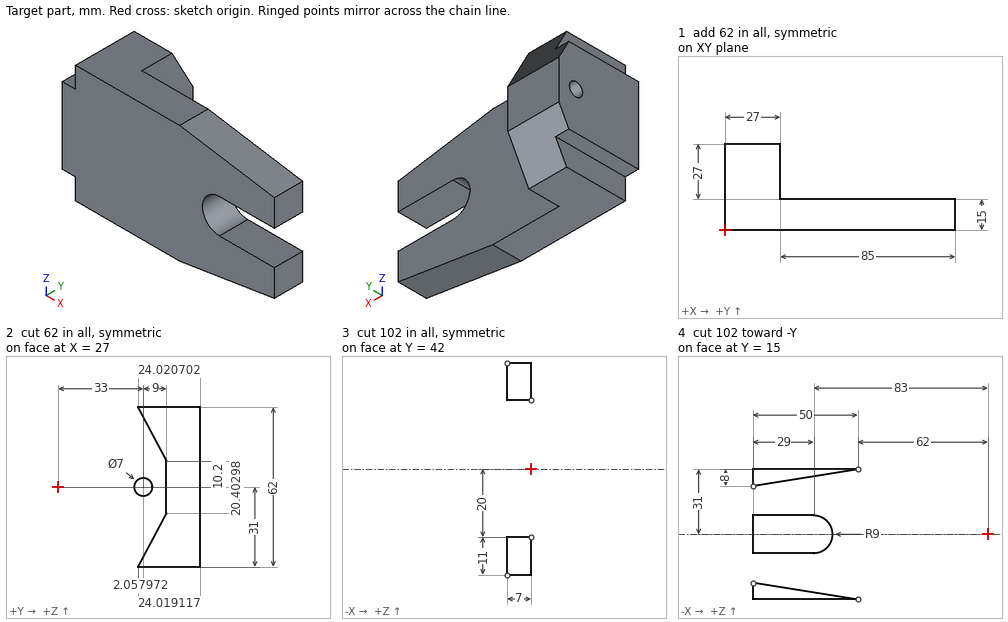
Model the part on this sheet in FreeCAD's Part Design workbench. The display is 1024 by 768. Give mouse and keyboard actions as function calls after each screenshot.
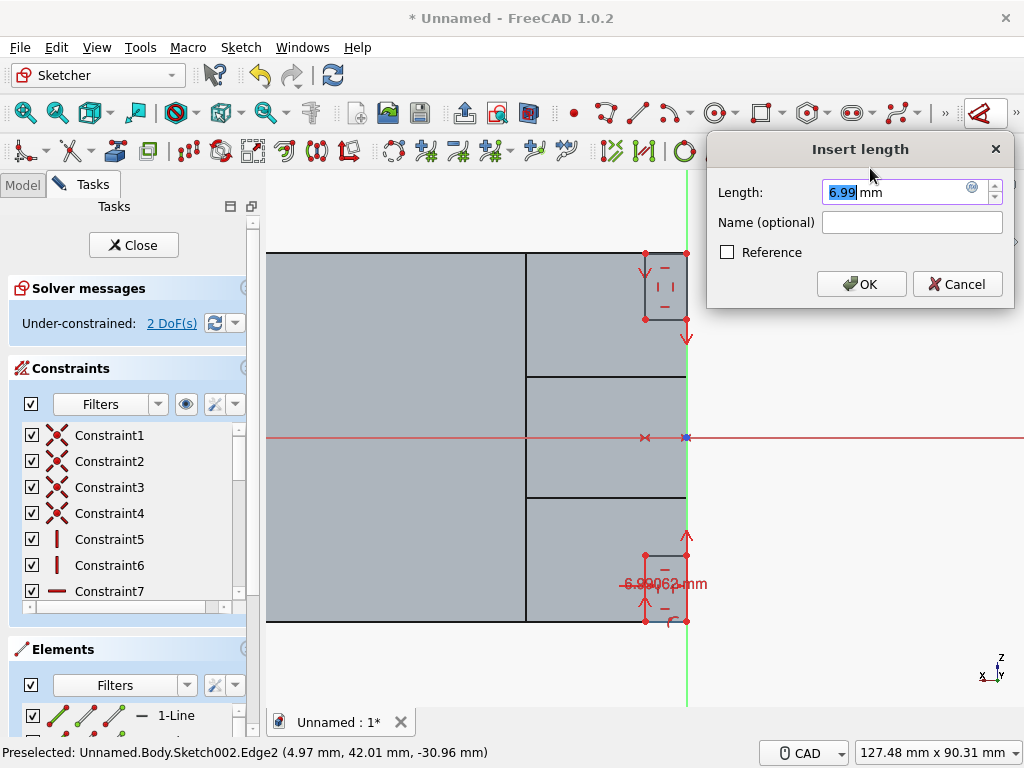
text(7)
key(Return)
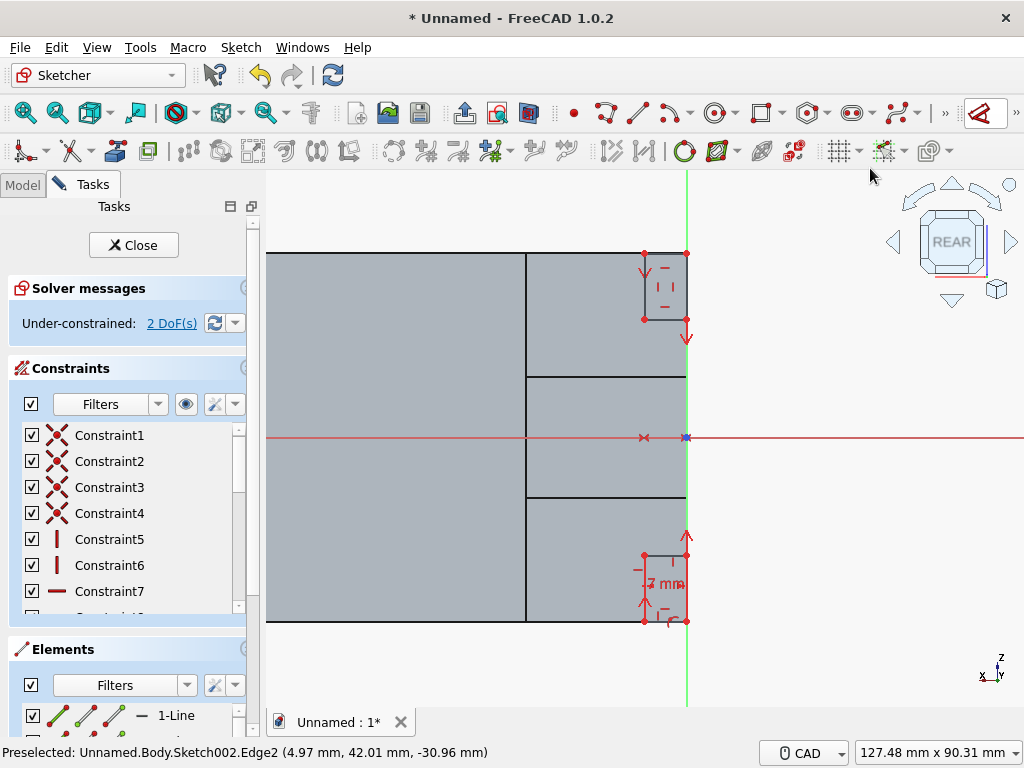
click(645, 576)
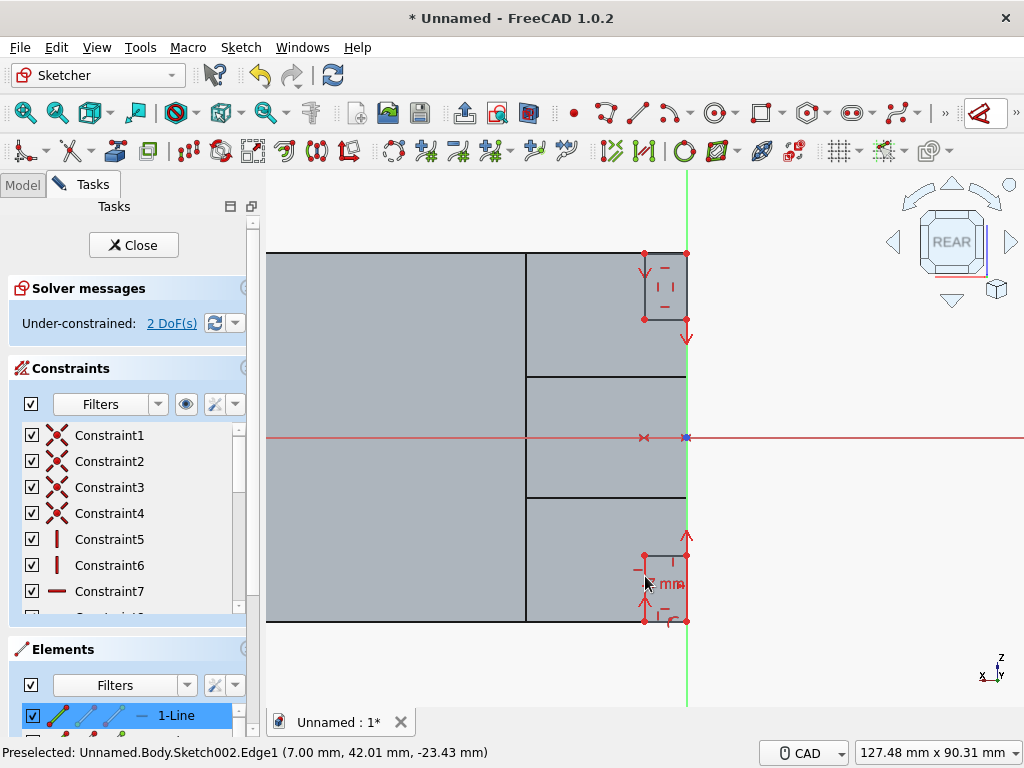
key(i)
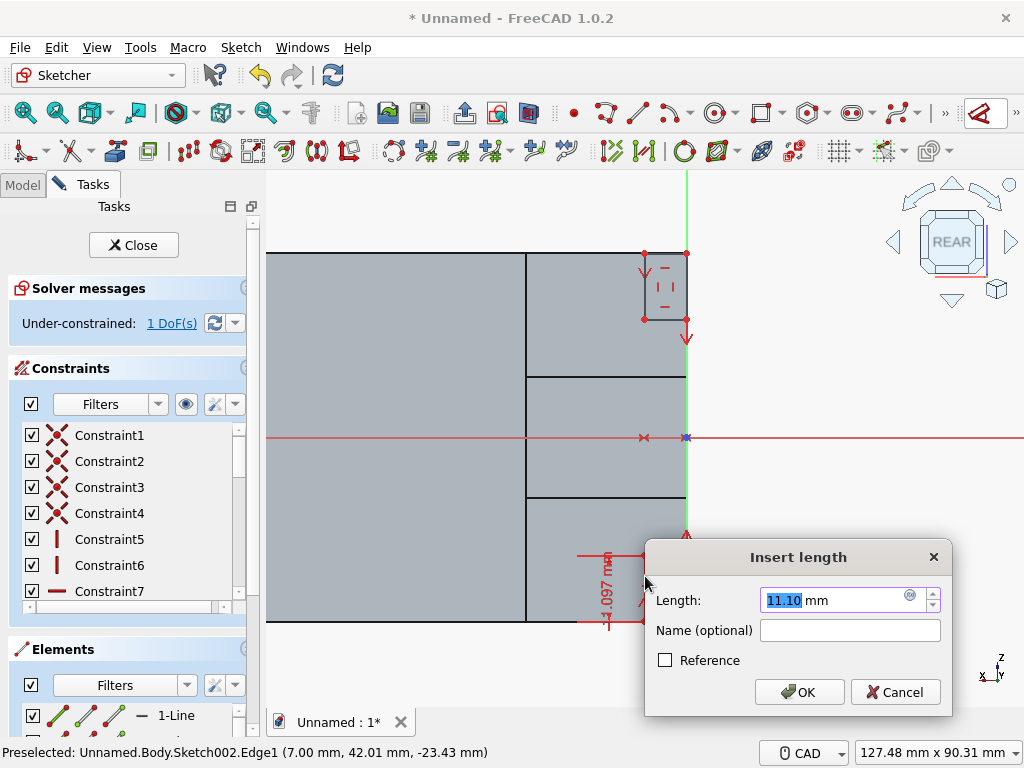
text(11)
key(Return)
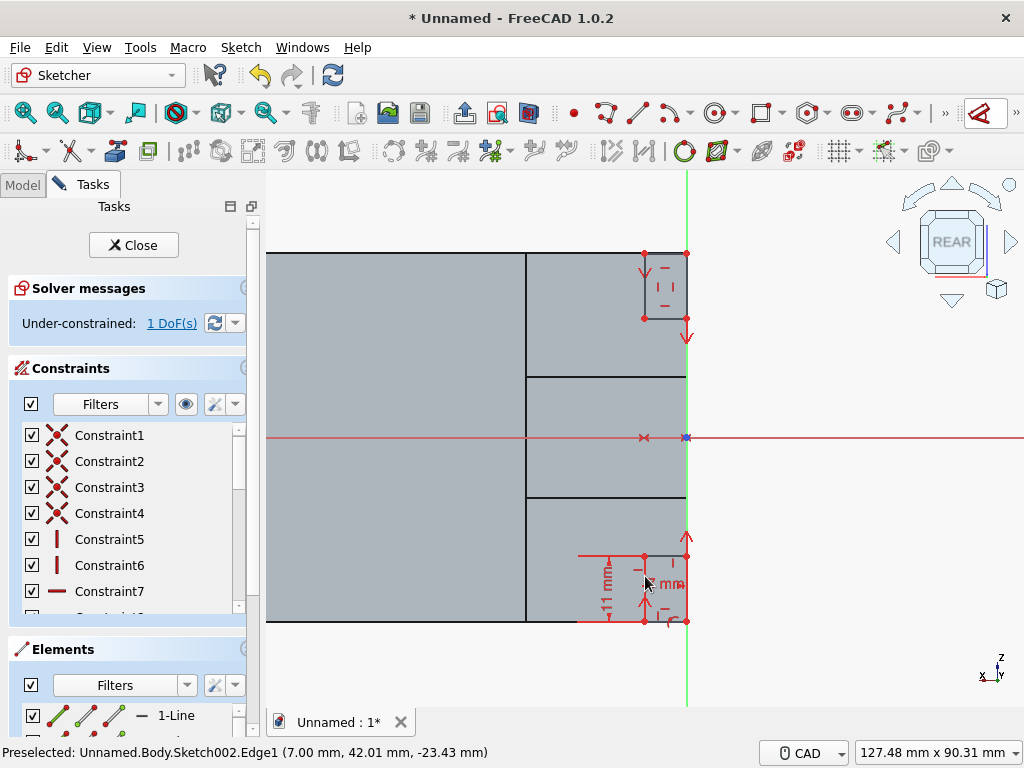
click(645, 556)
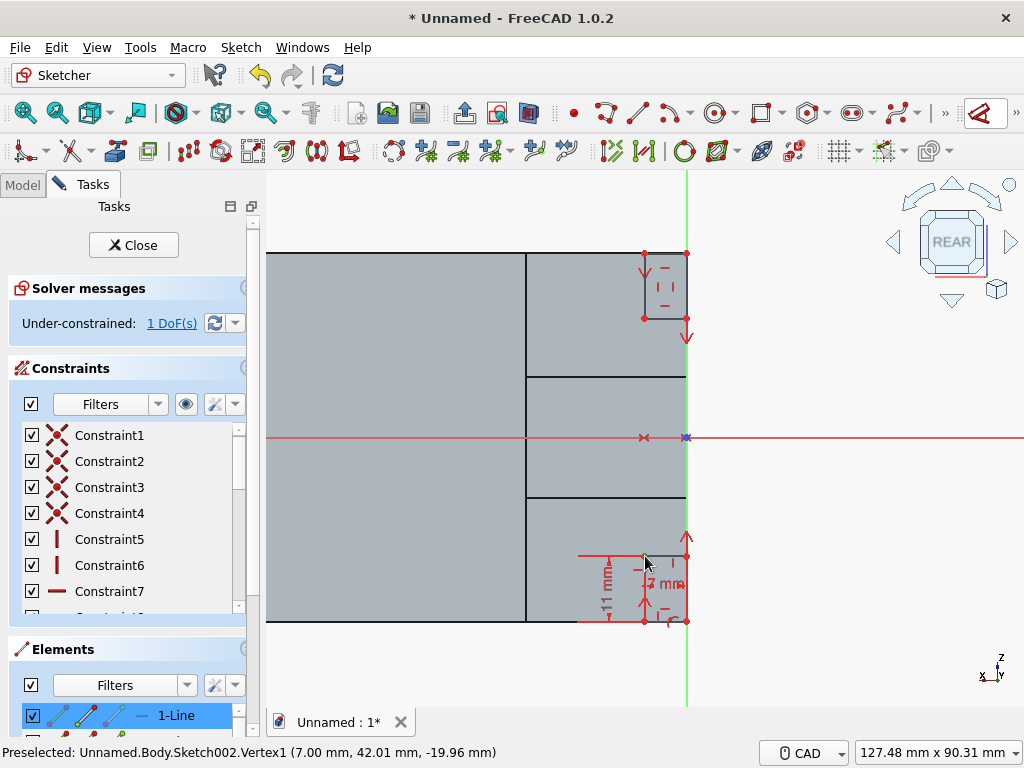
key(i)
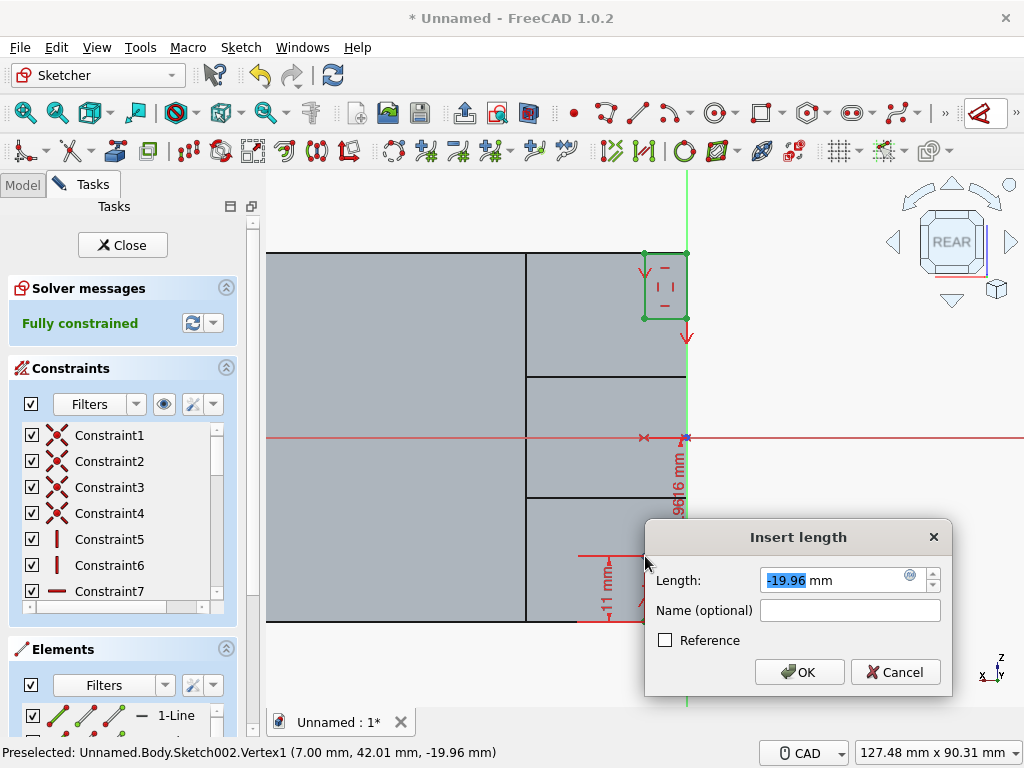
text(-20)
key(Return)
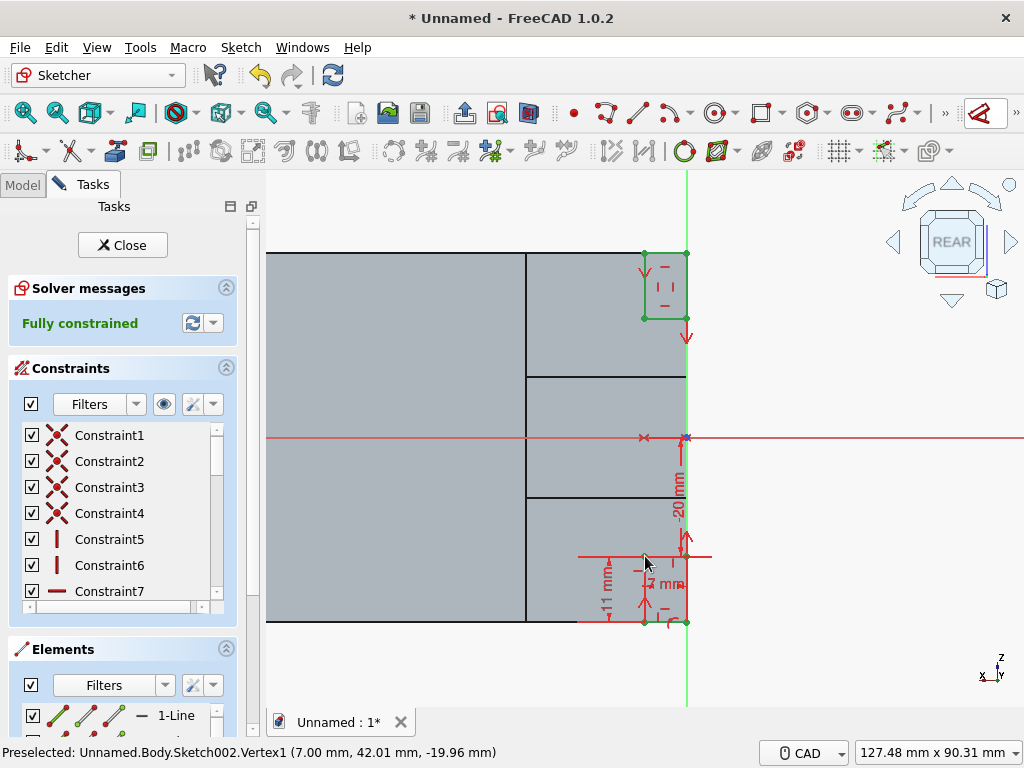
click(123, 245)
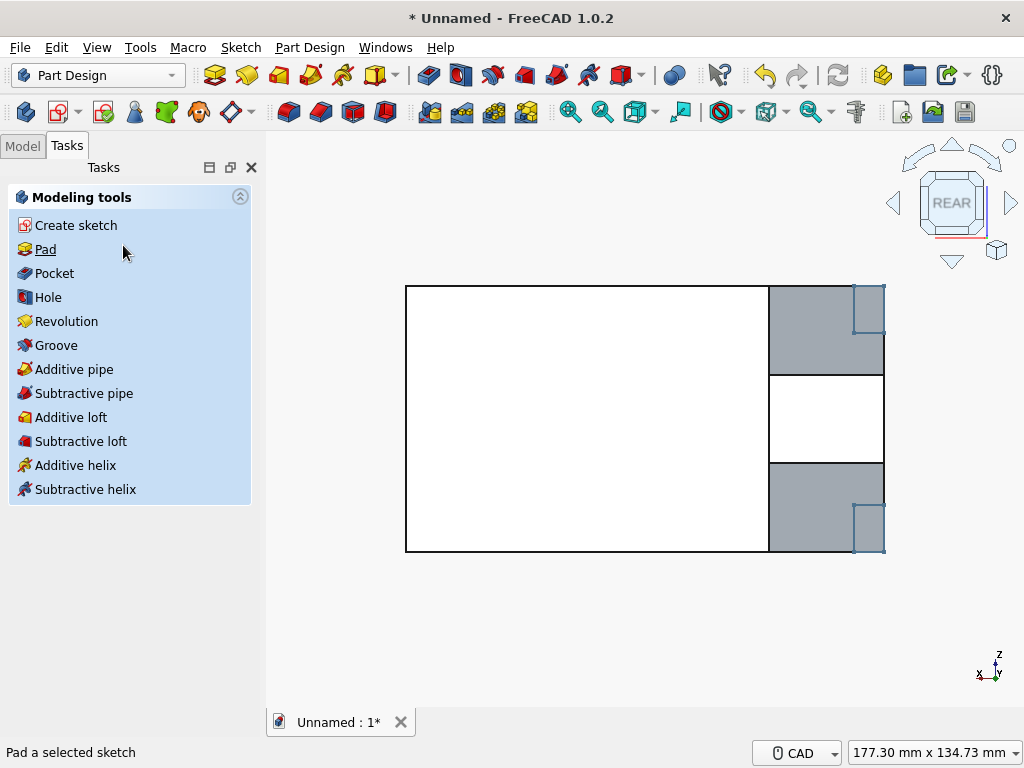
click(430, 76)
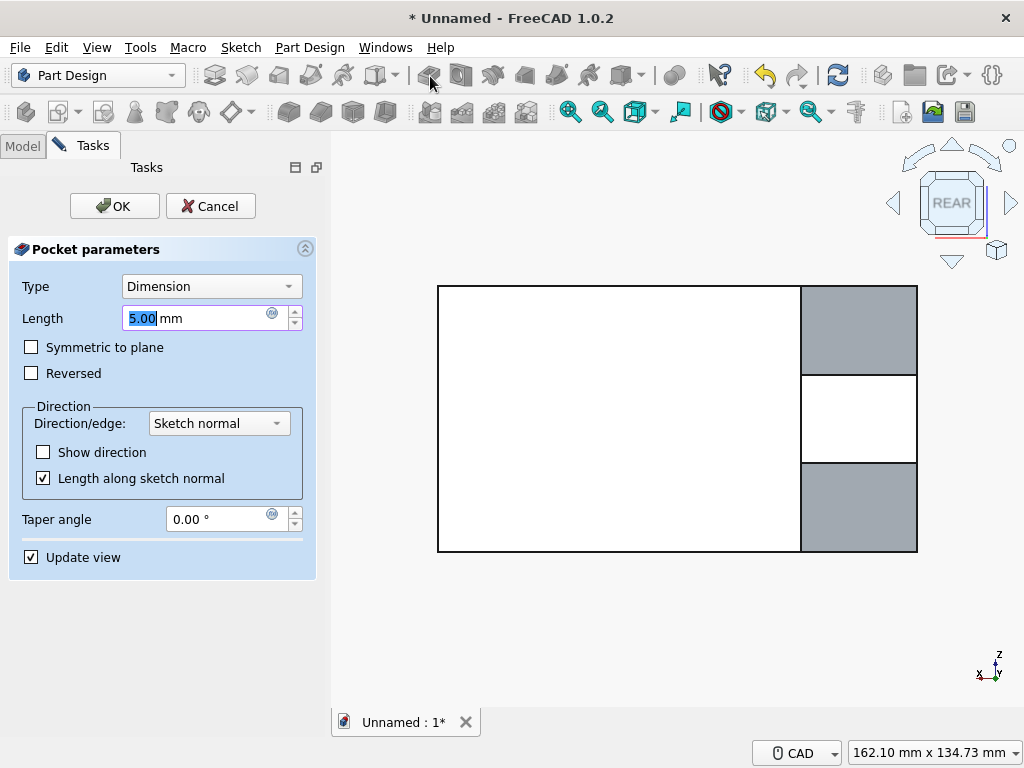
text(102)
key(Tab)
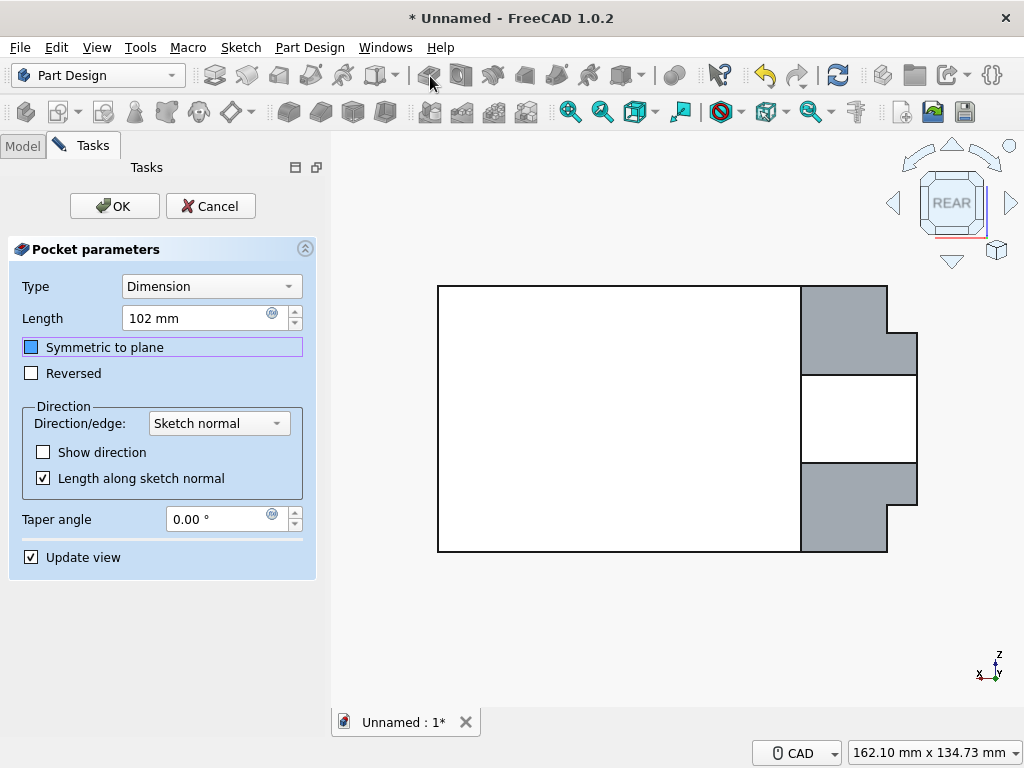
click(30, 347)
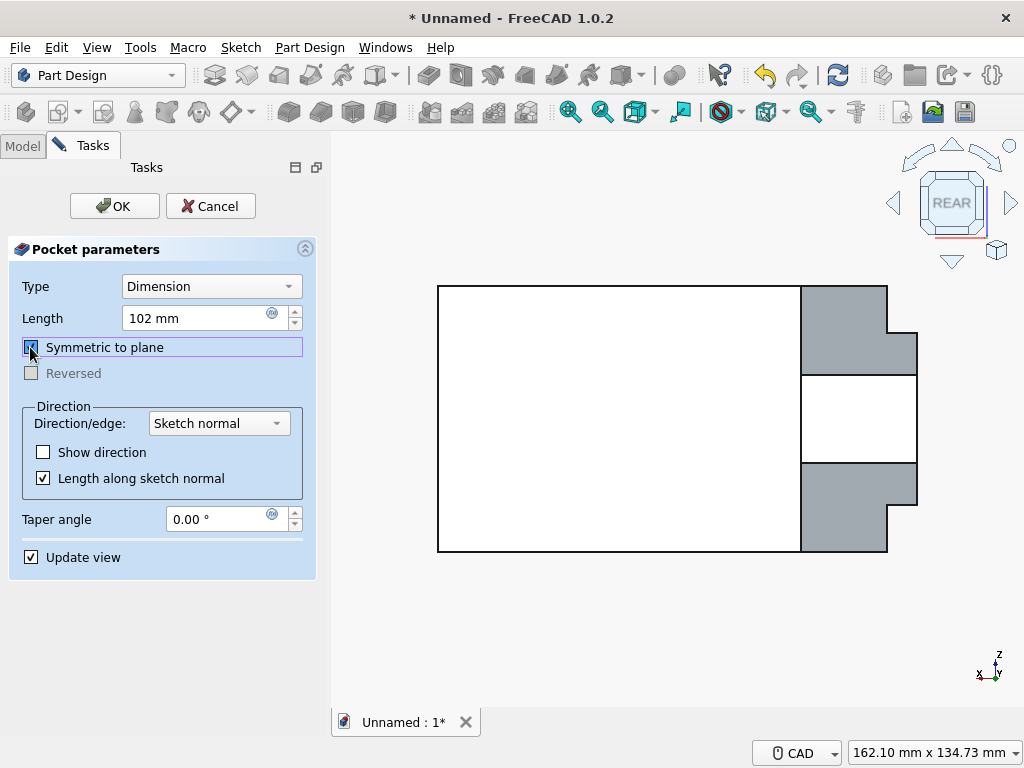
click(115, 206)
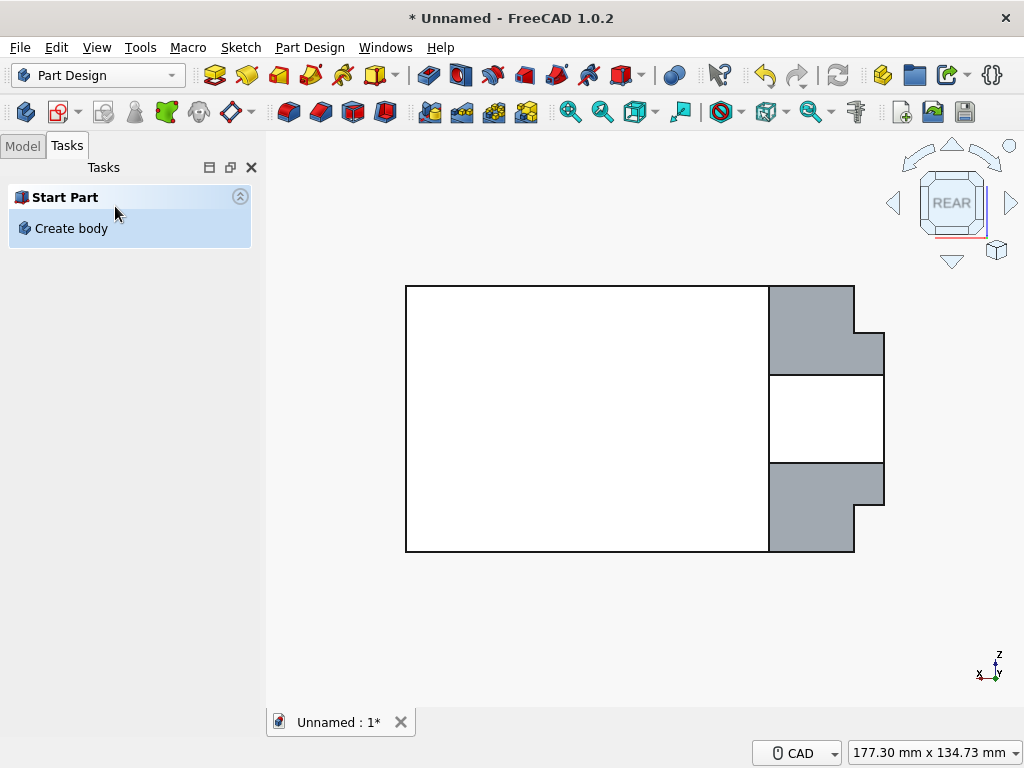
click(587, 418)